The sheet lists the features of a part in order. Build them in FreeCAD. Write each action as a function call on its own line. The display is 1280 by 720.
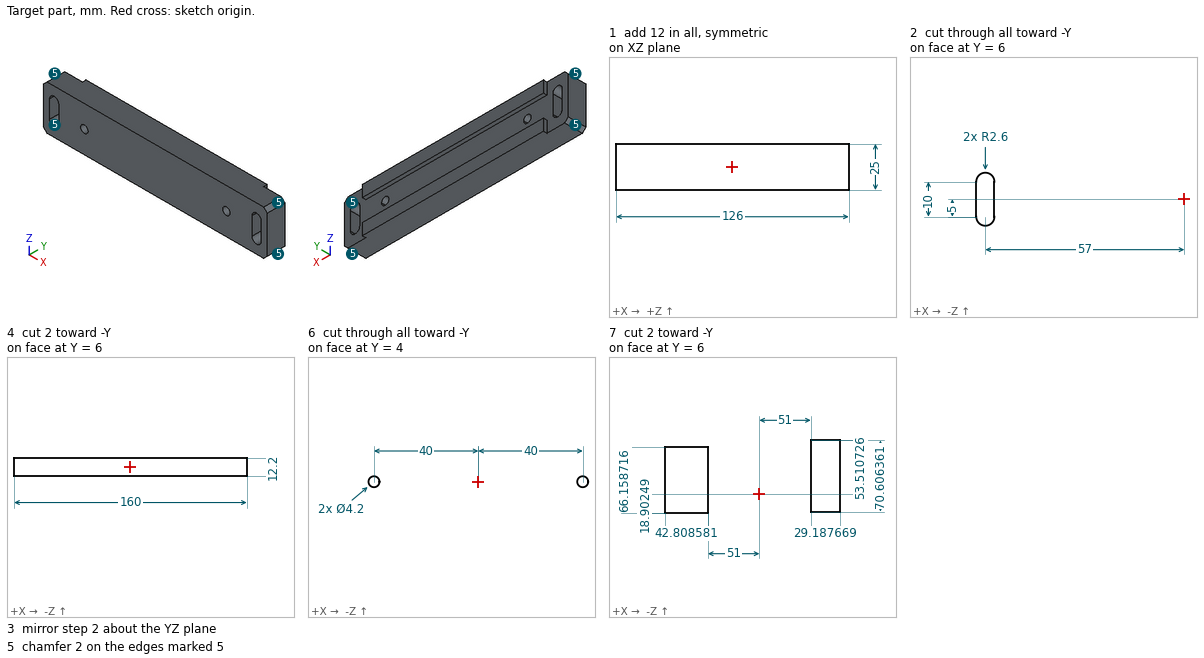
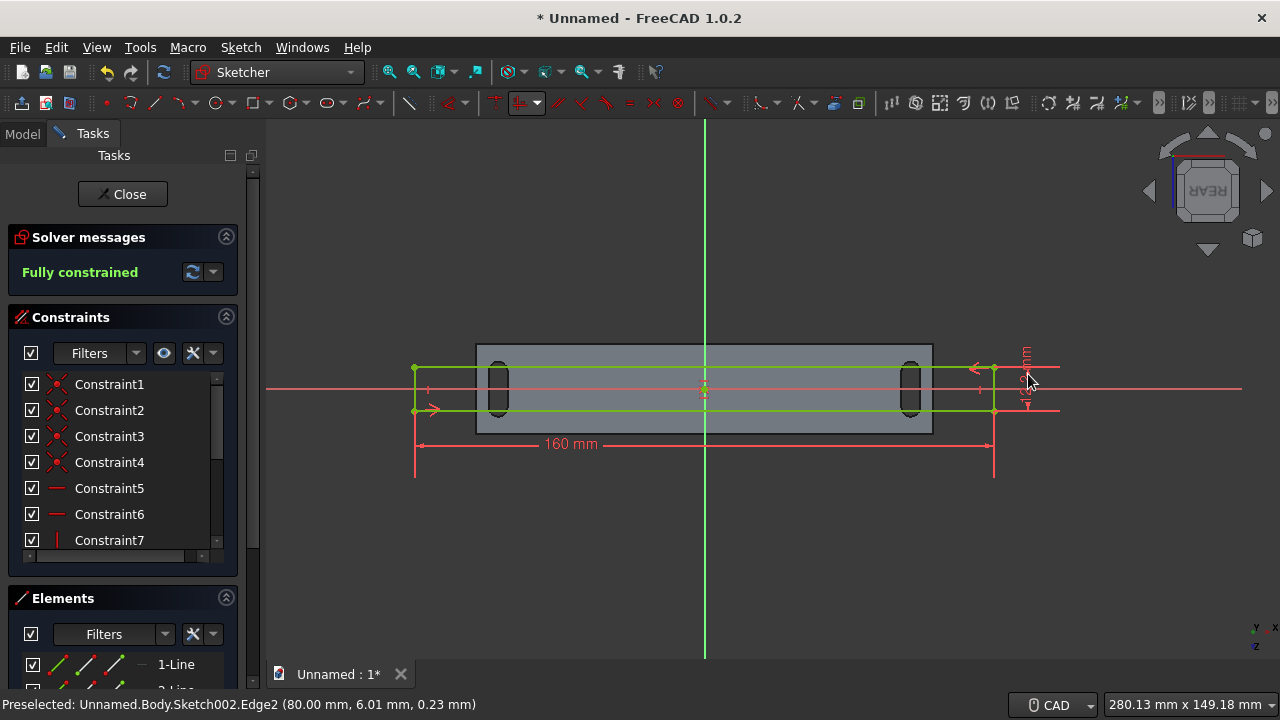
click(123, 194)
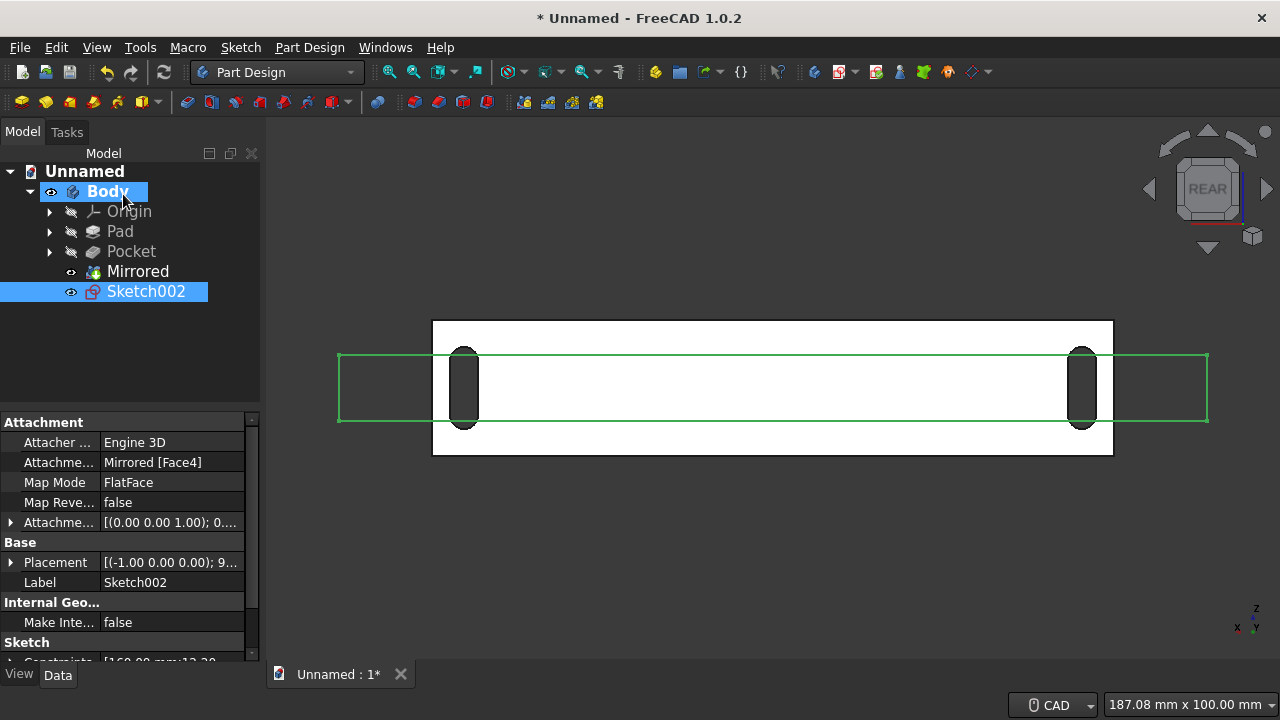
click(188, 102)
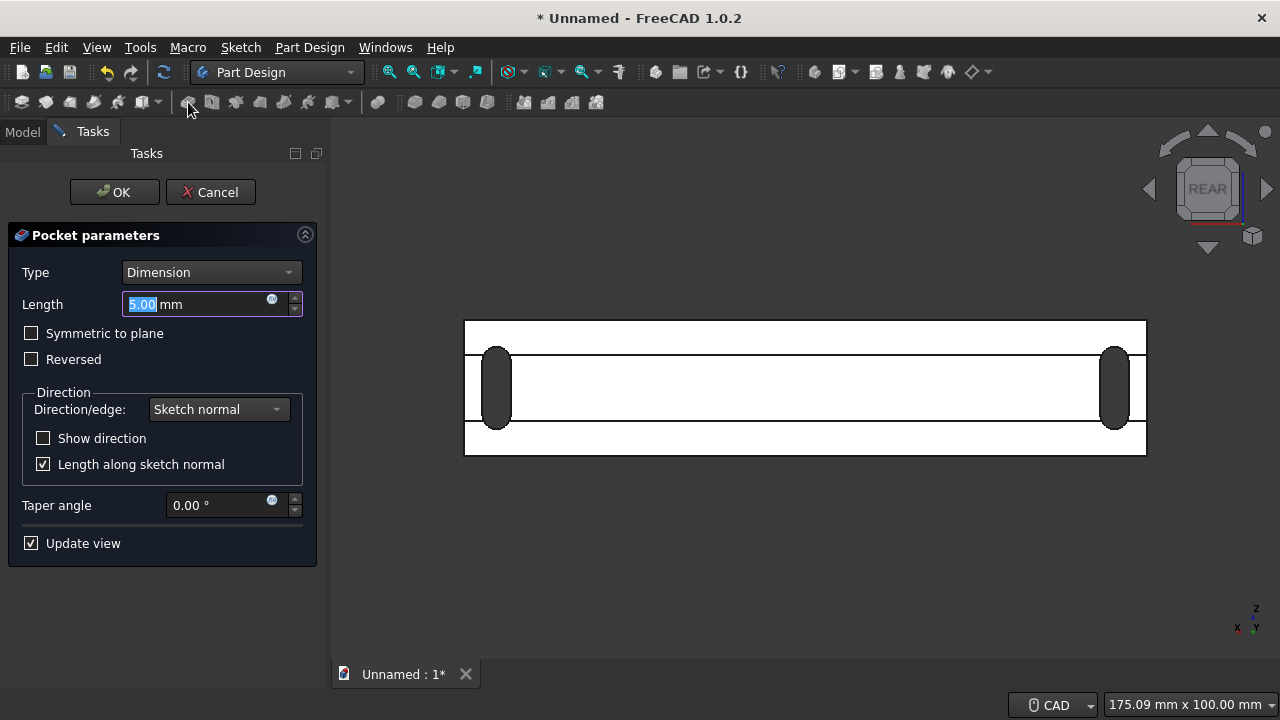
text(2)
key(Tab)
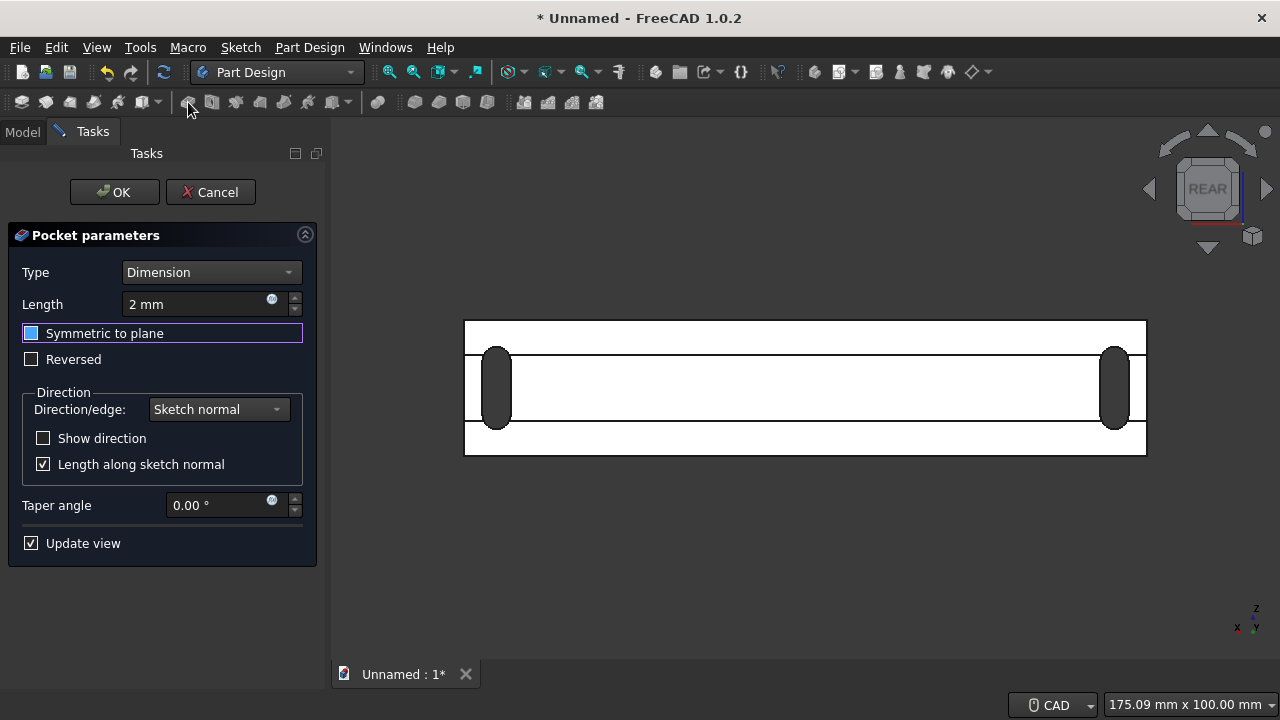
click(115, 192)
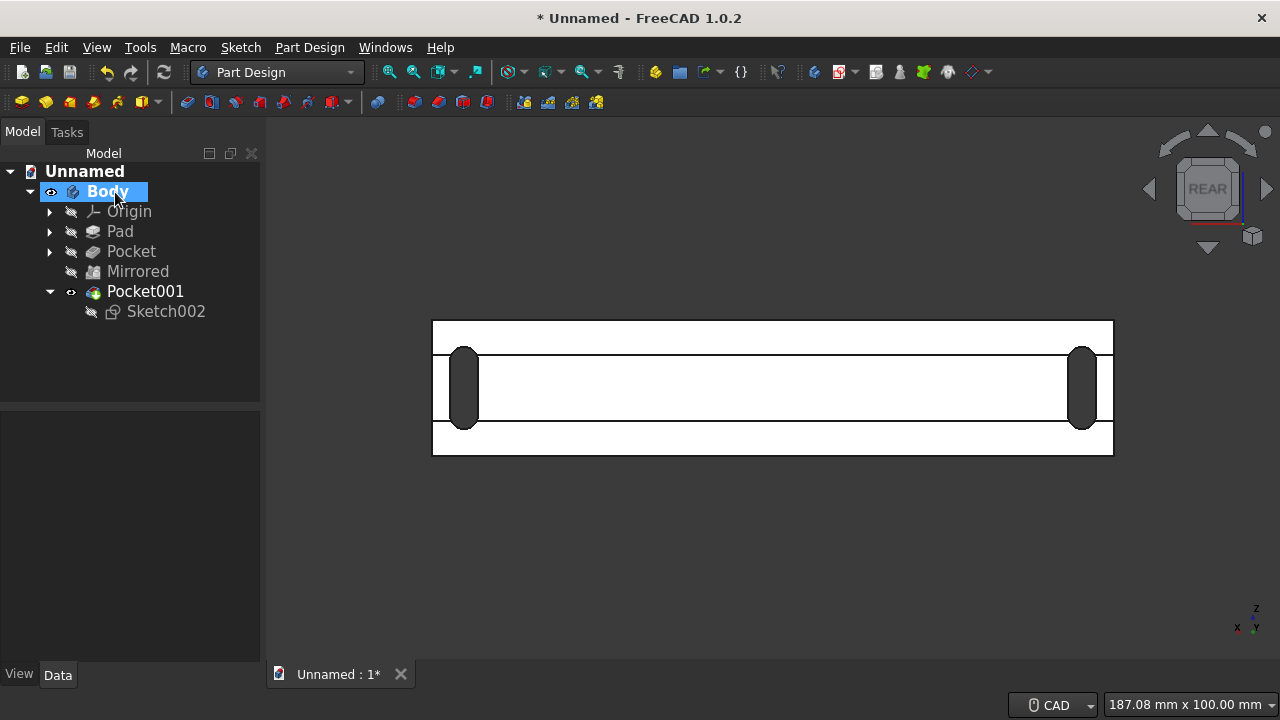
key(0)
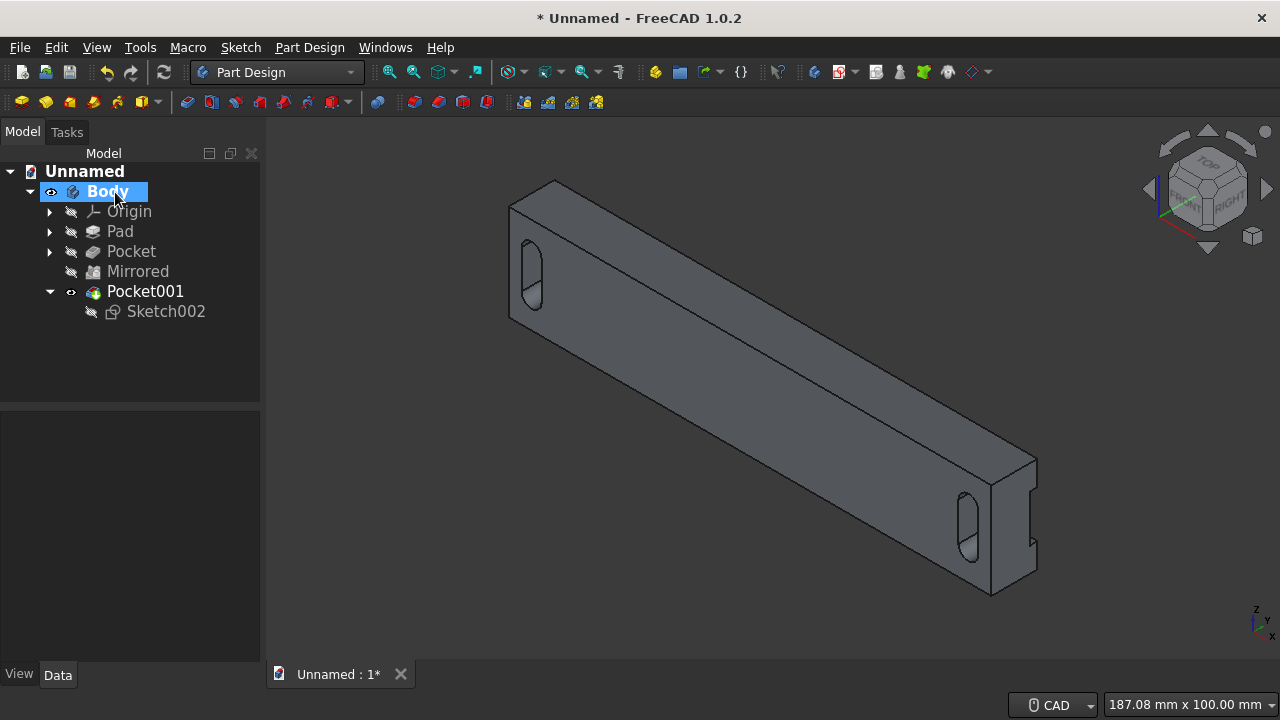
click(1014, 471)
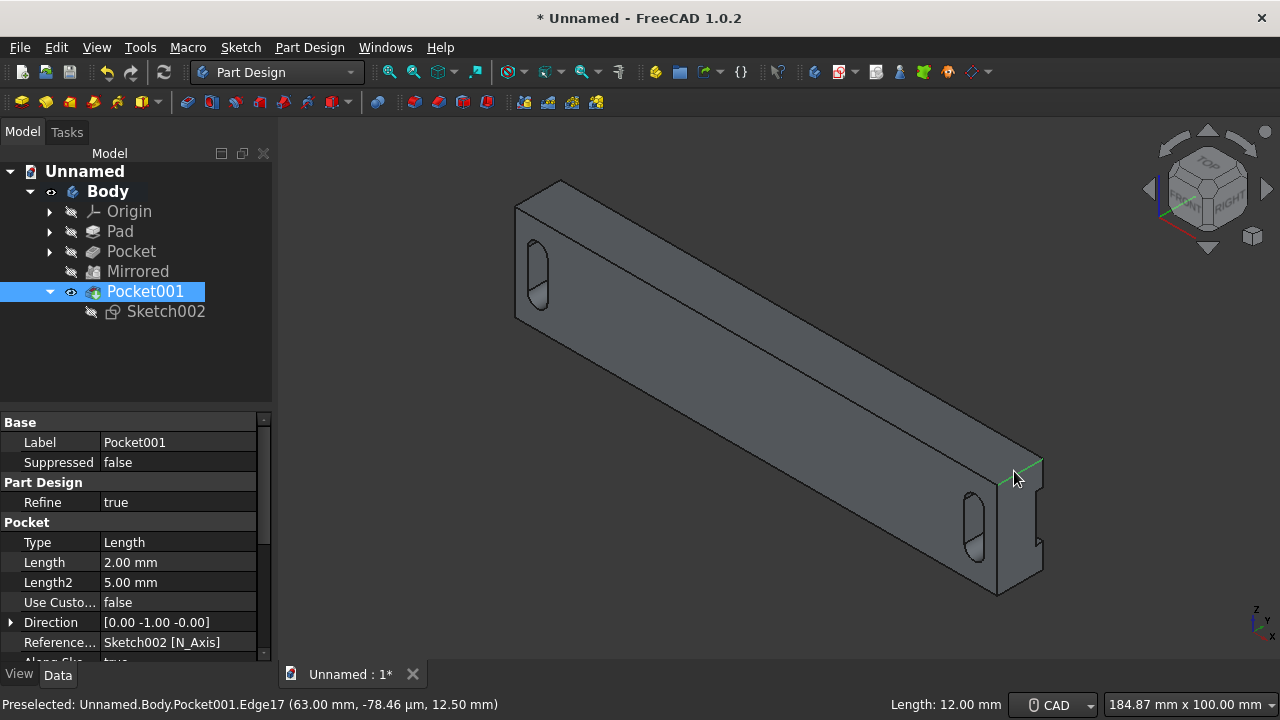
key(2)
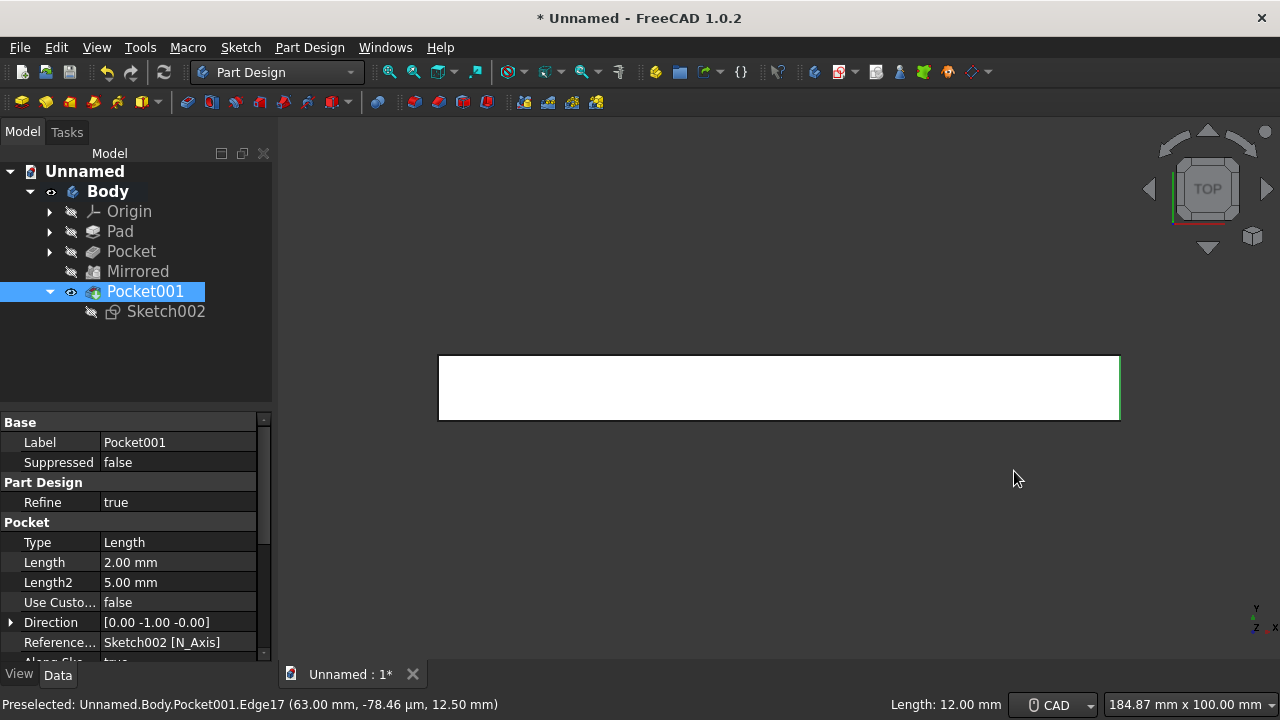
click(438, 387, ctrl)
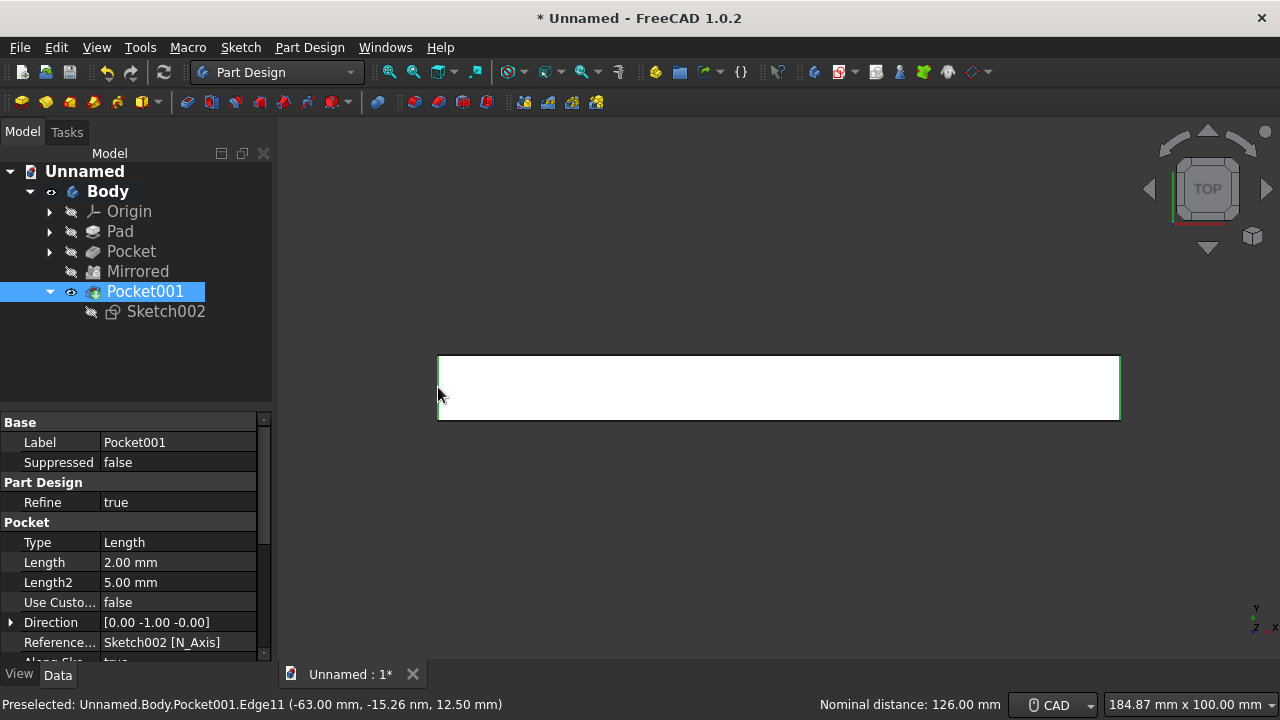
key(1)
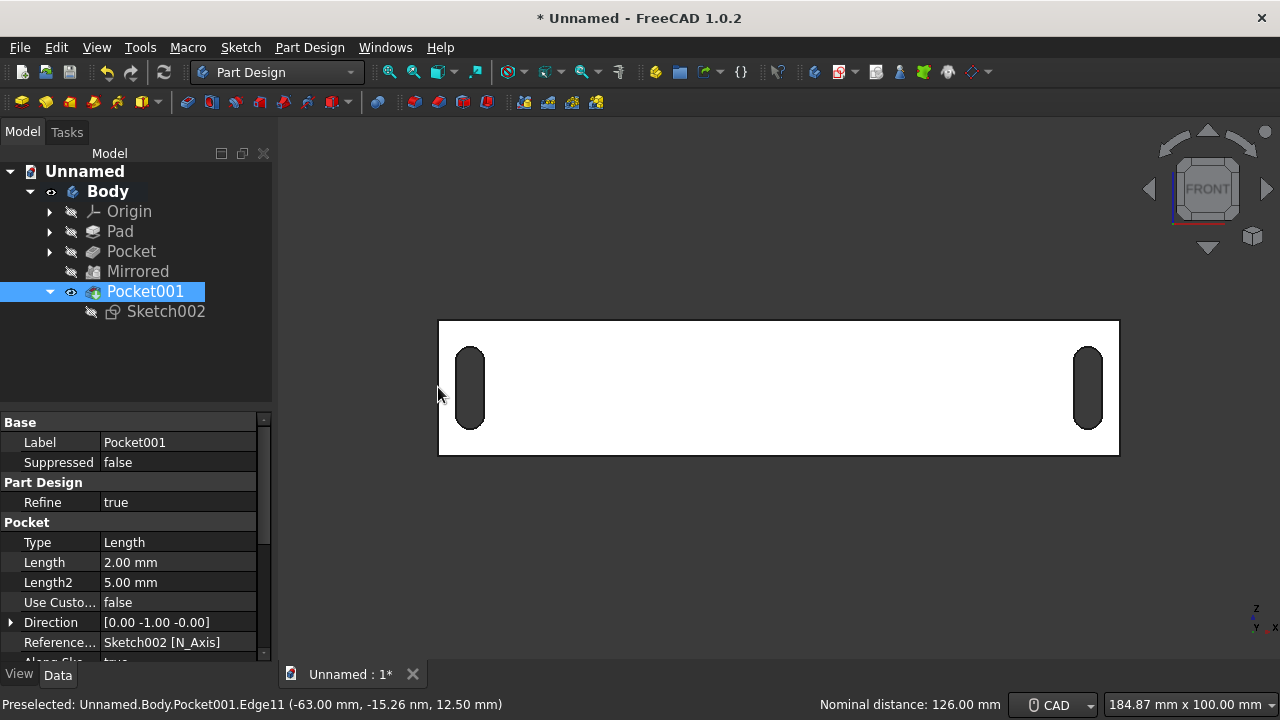
key(3)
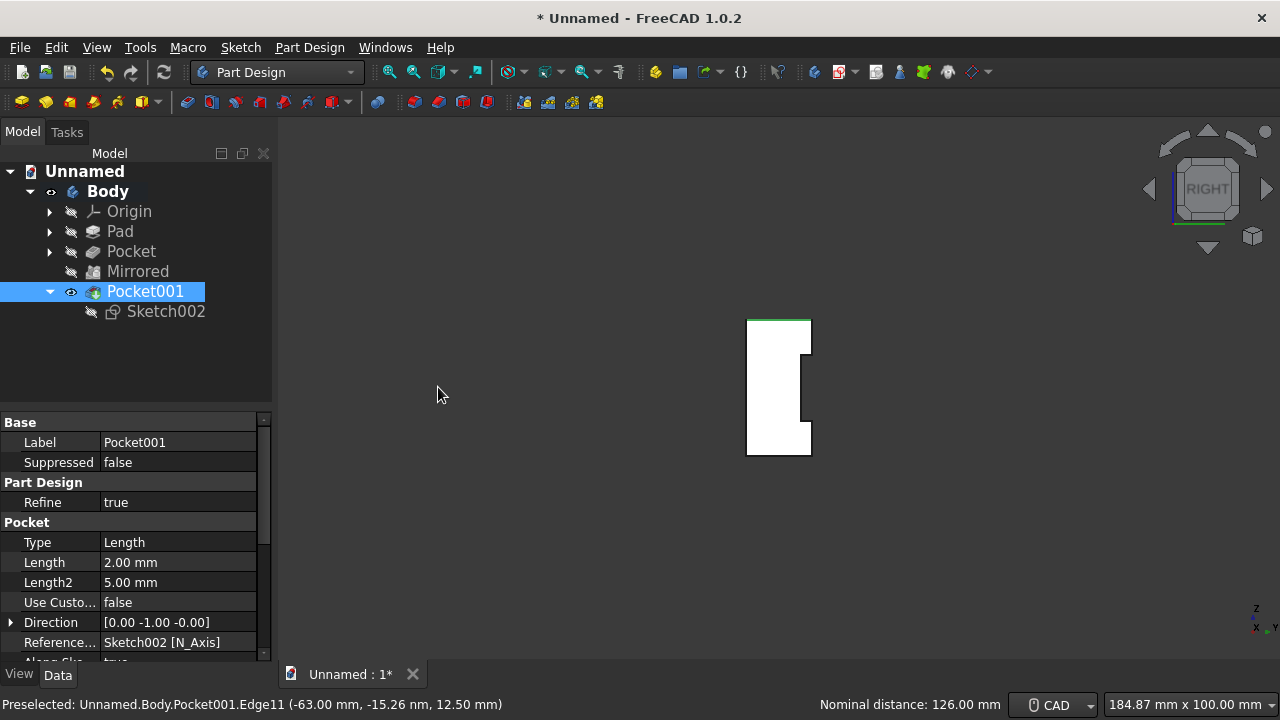
click(390, 72)